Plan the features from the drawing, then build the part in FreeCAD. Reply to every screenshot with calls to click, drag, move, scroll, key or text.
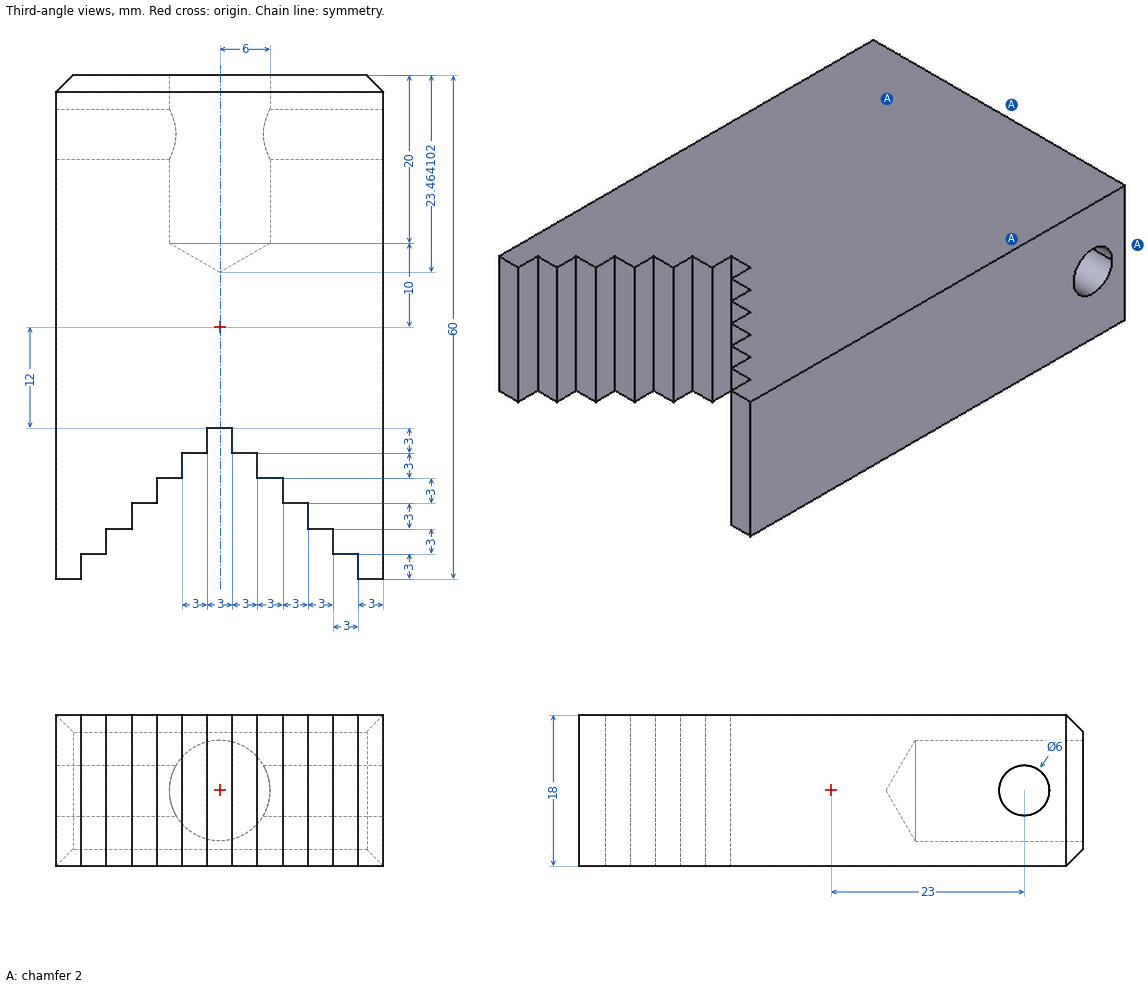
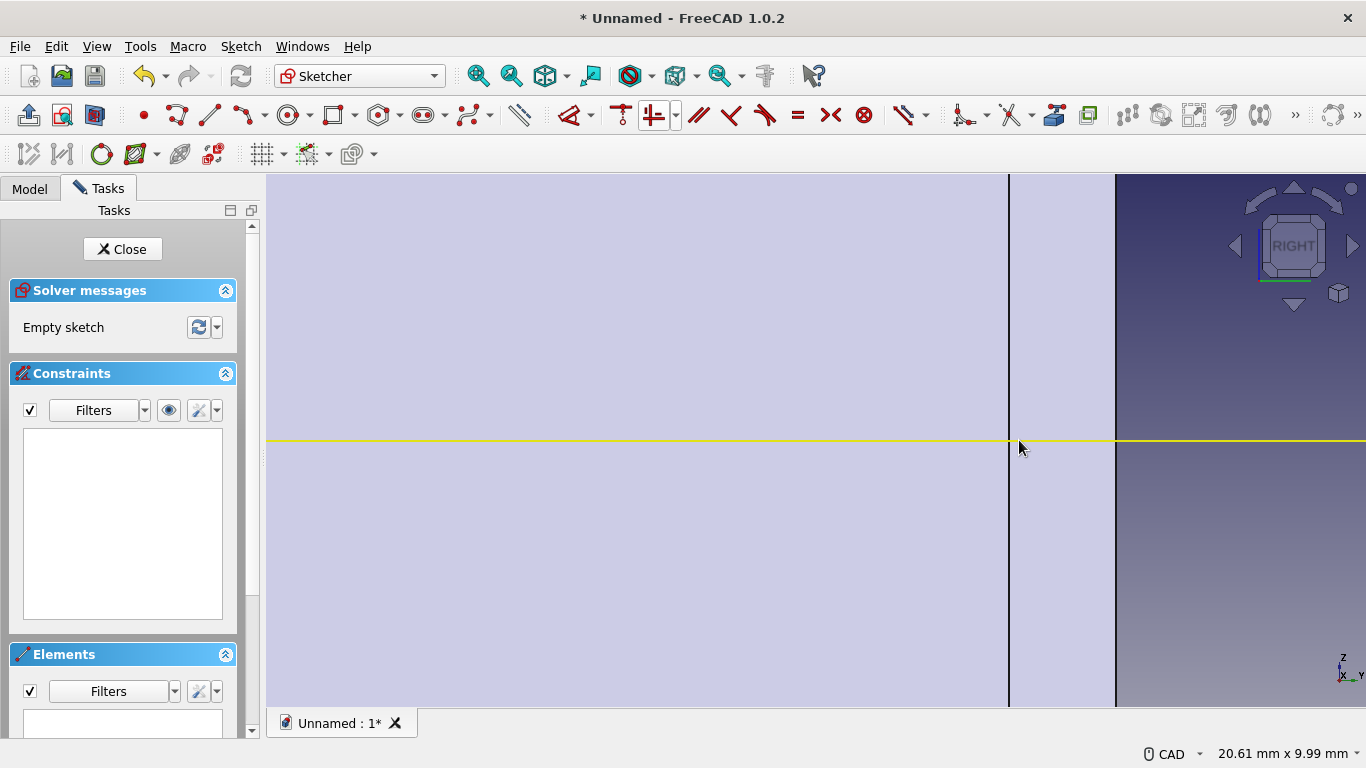
key(g)
key(c)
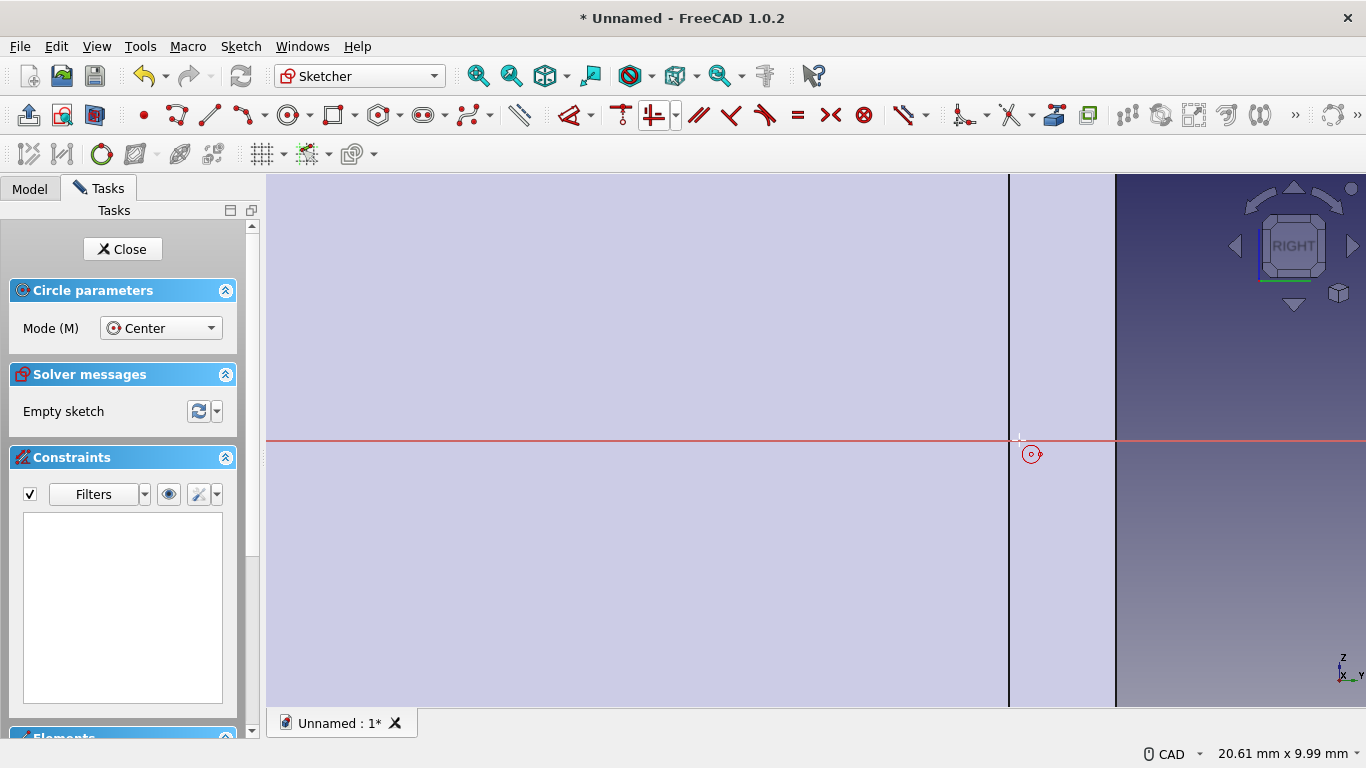
click(742, 440)
click(855, 327)
key(Escape)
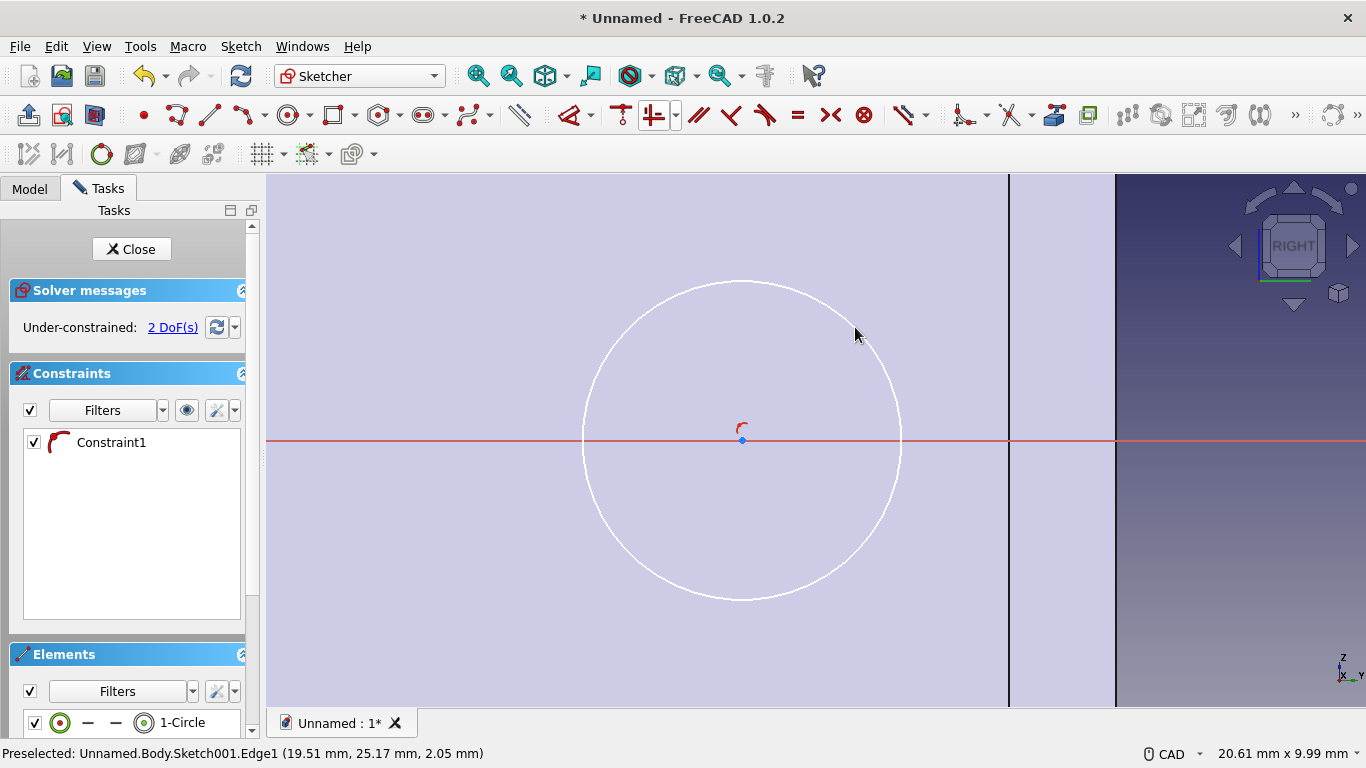
key(d)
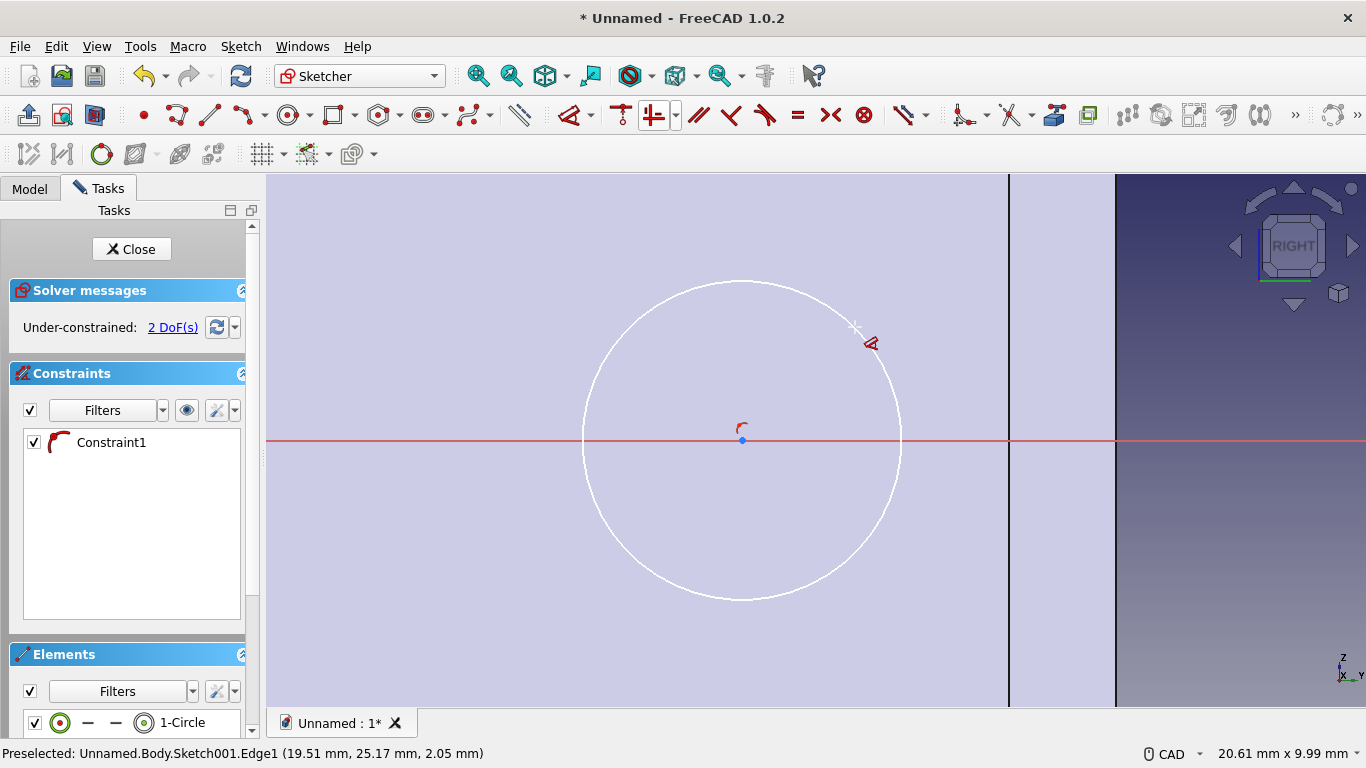
click(854, 327)
click(876, 304)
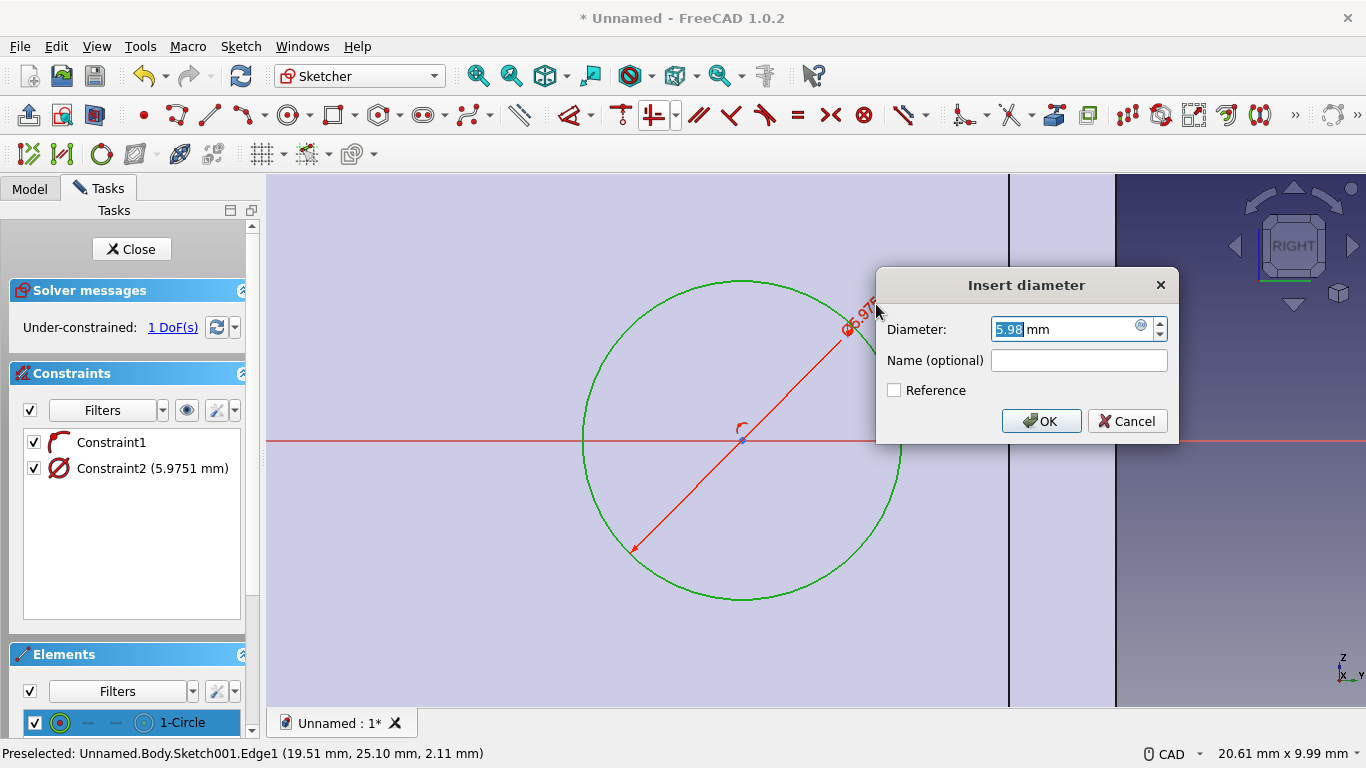
text(6)
key(Return)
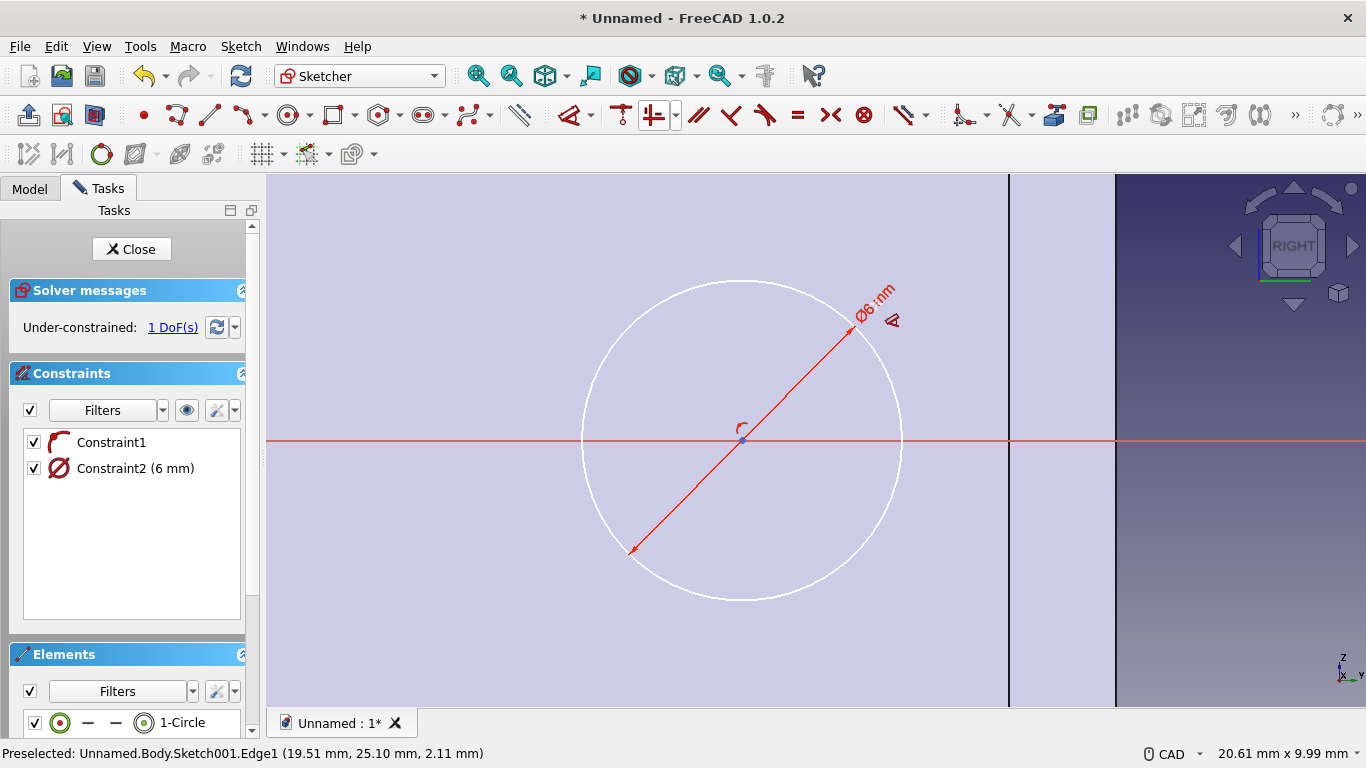
click(742, 440)
click(518, 474)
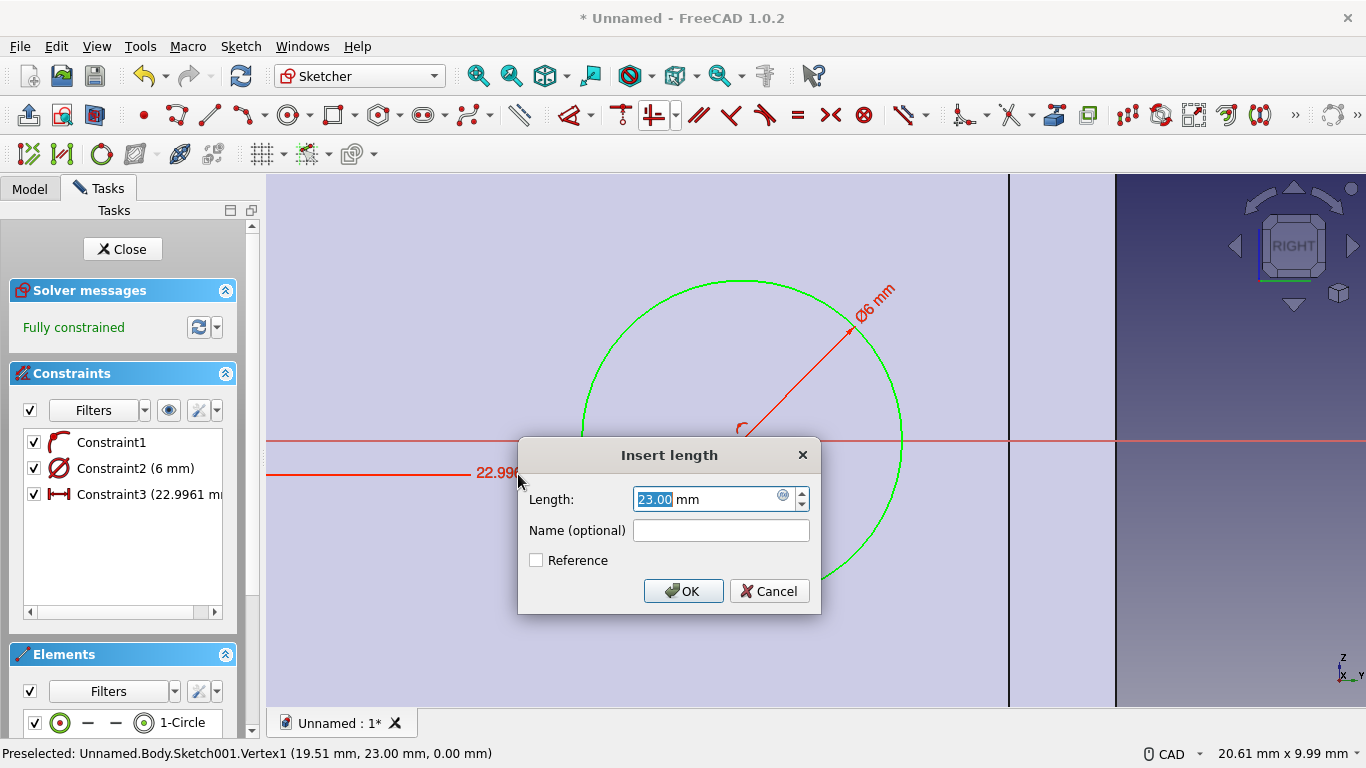
text(23)
key(Return)
key(Escape)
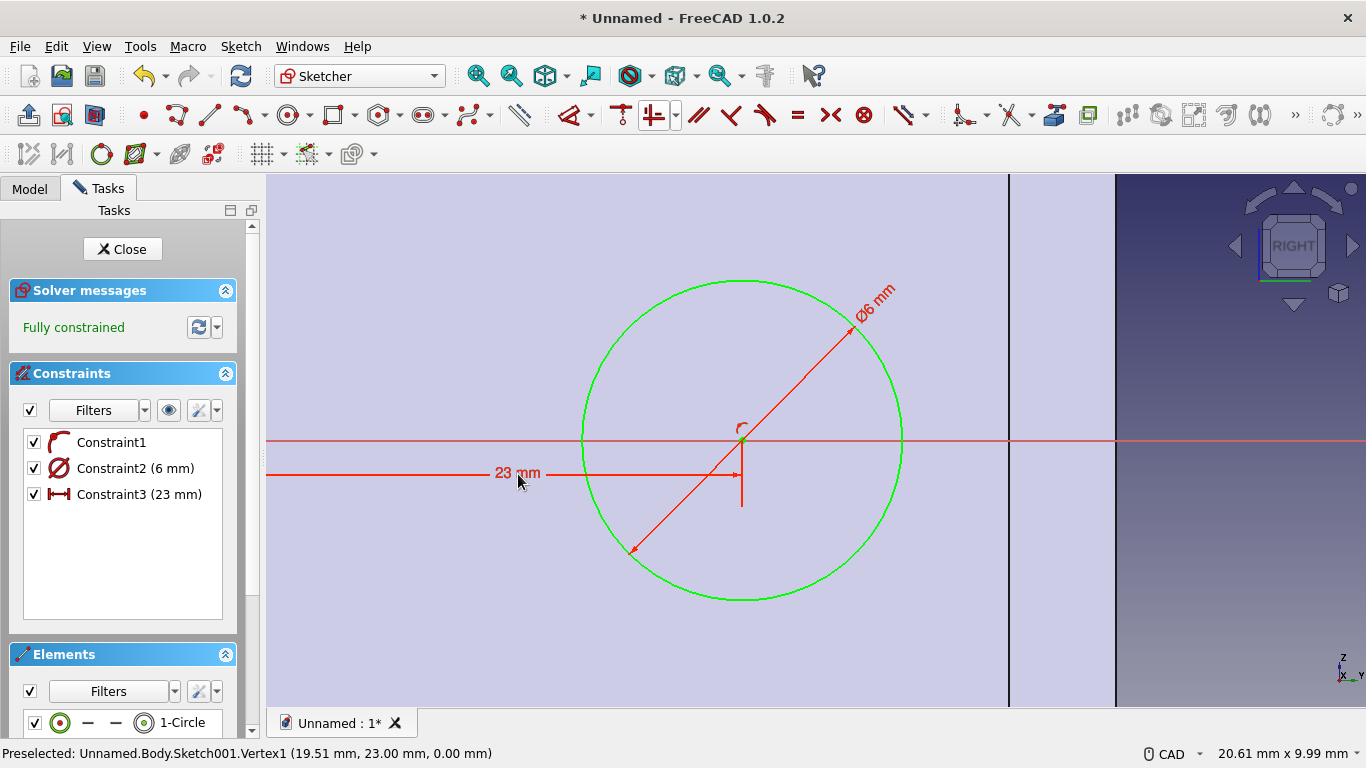
click(123, 249)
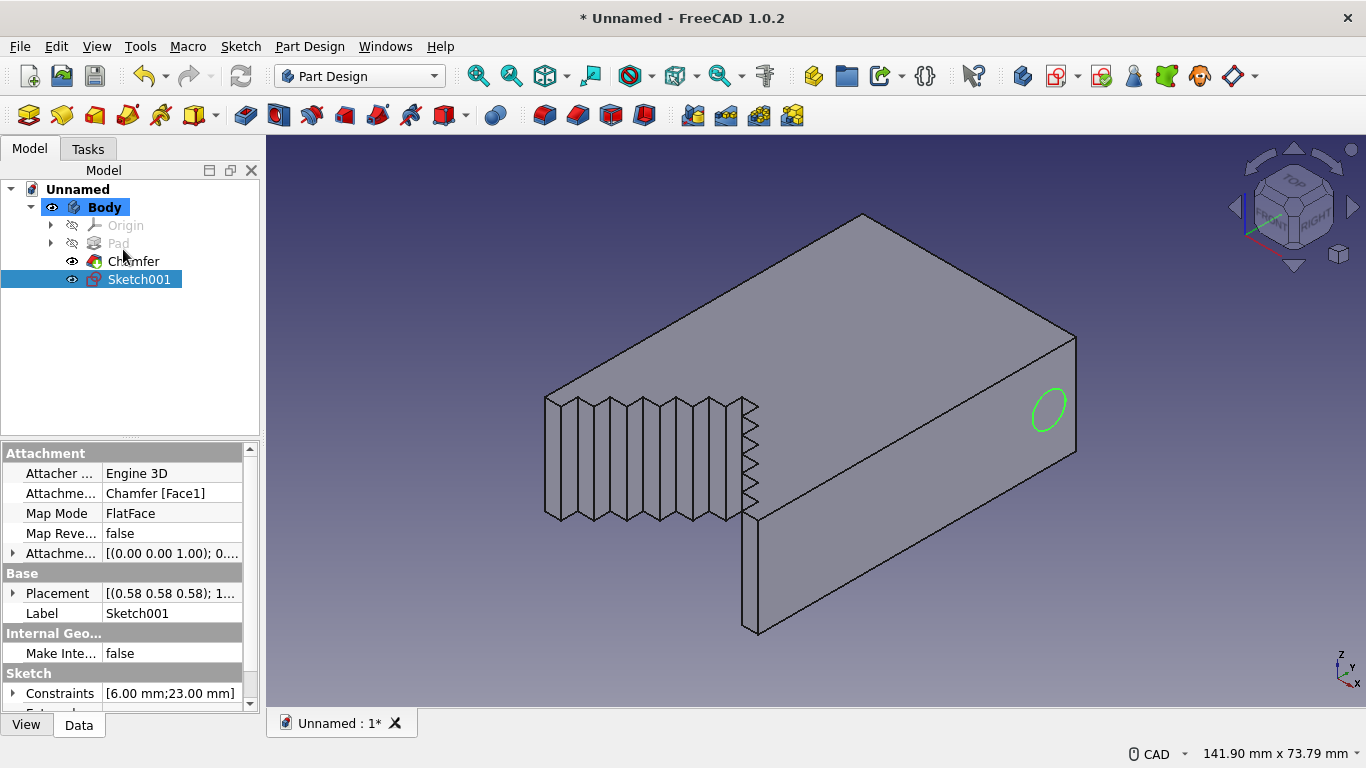
click(246, 116)